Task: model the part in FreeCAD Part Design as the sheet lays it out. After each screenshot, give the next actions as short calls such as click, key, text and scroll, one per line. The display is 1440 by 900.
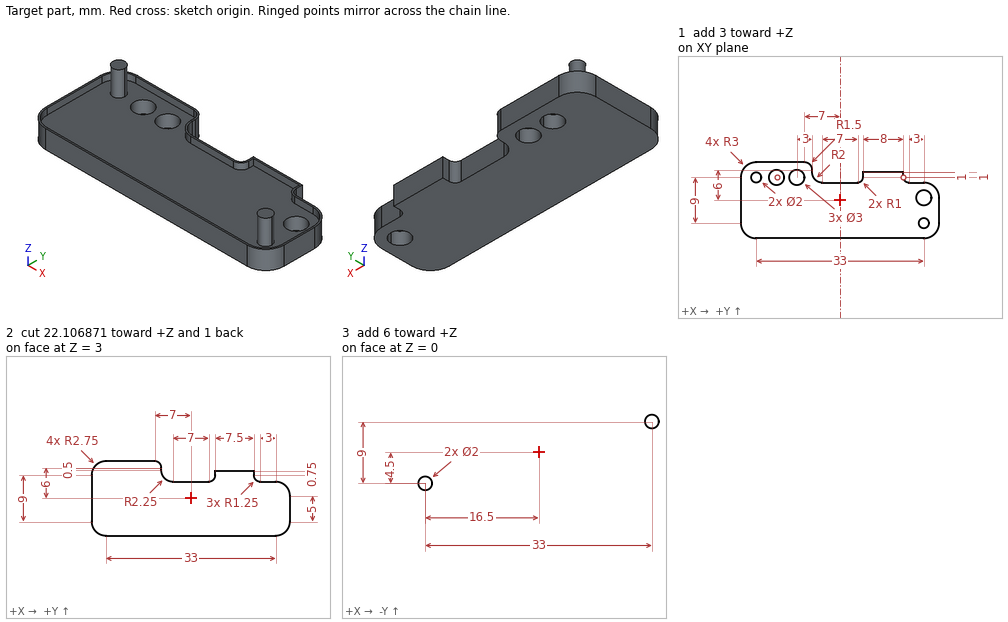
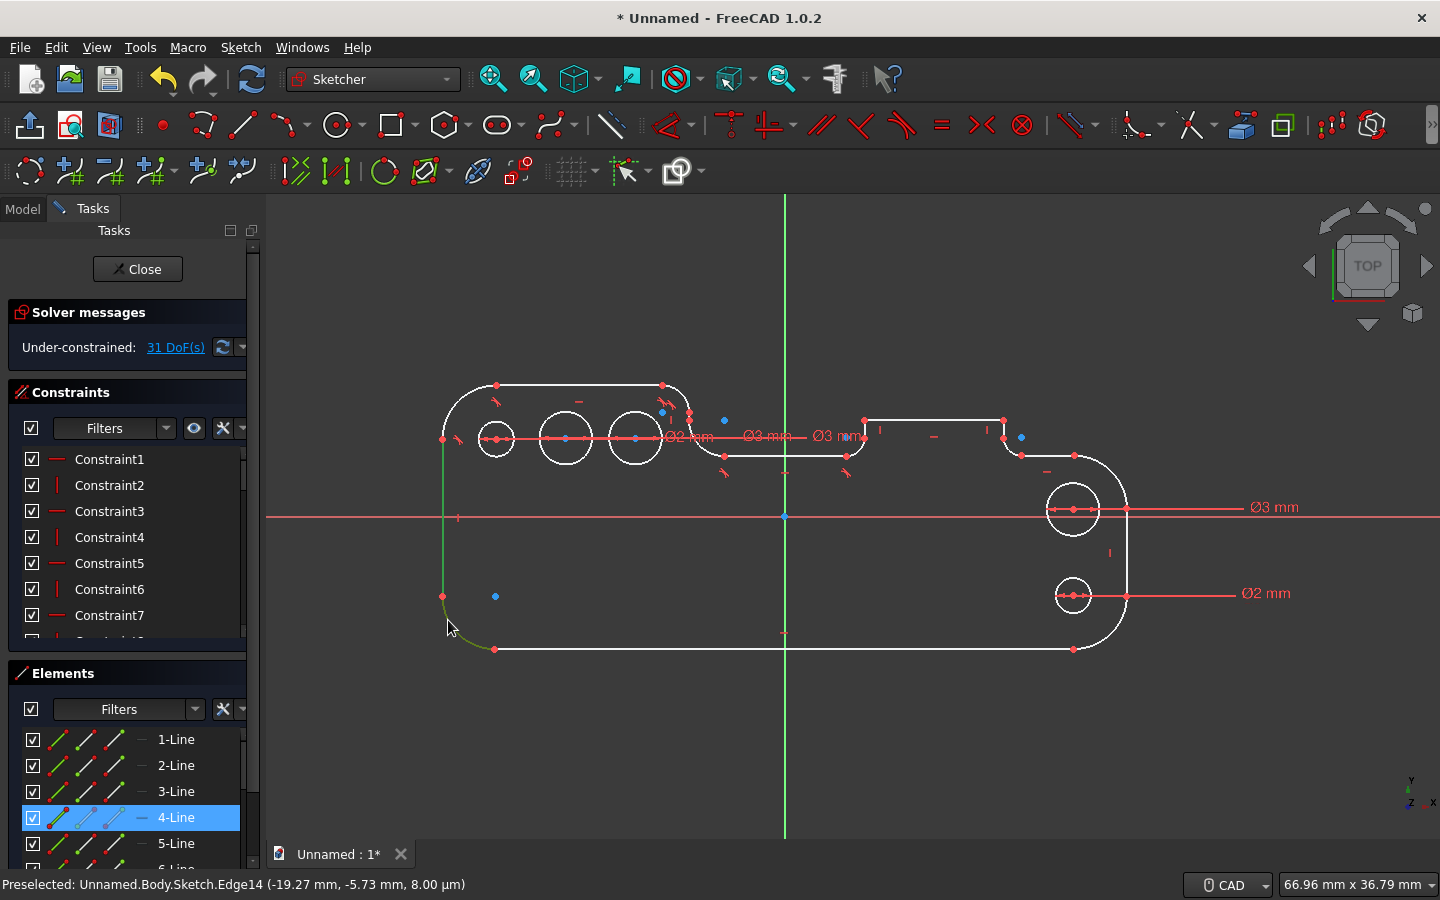
key(t)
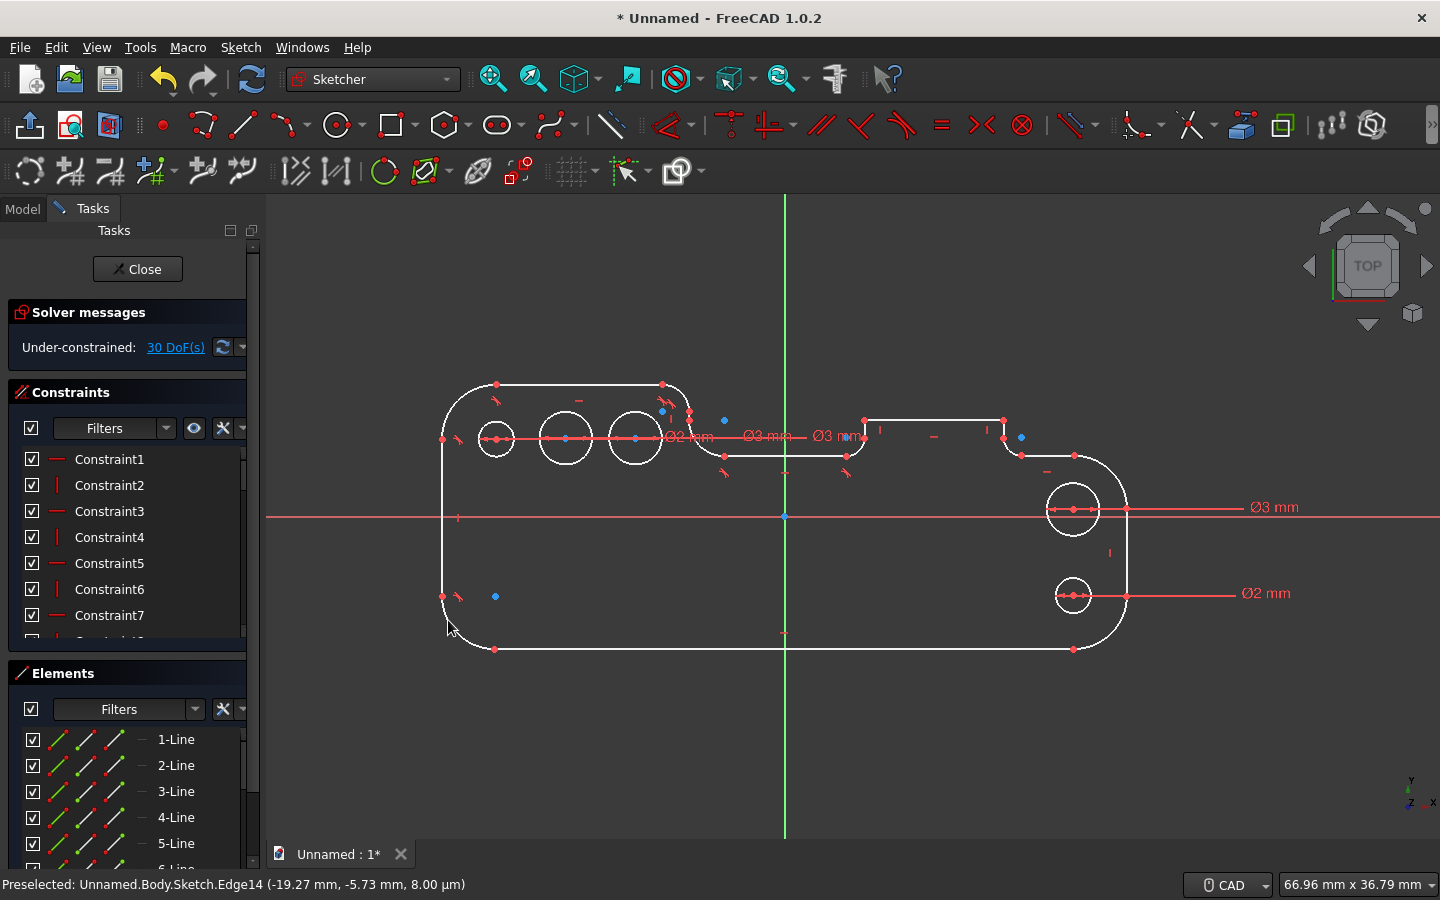
click(669, 649)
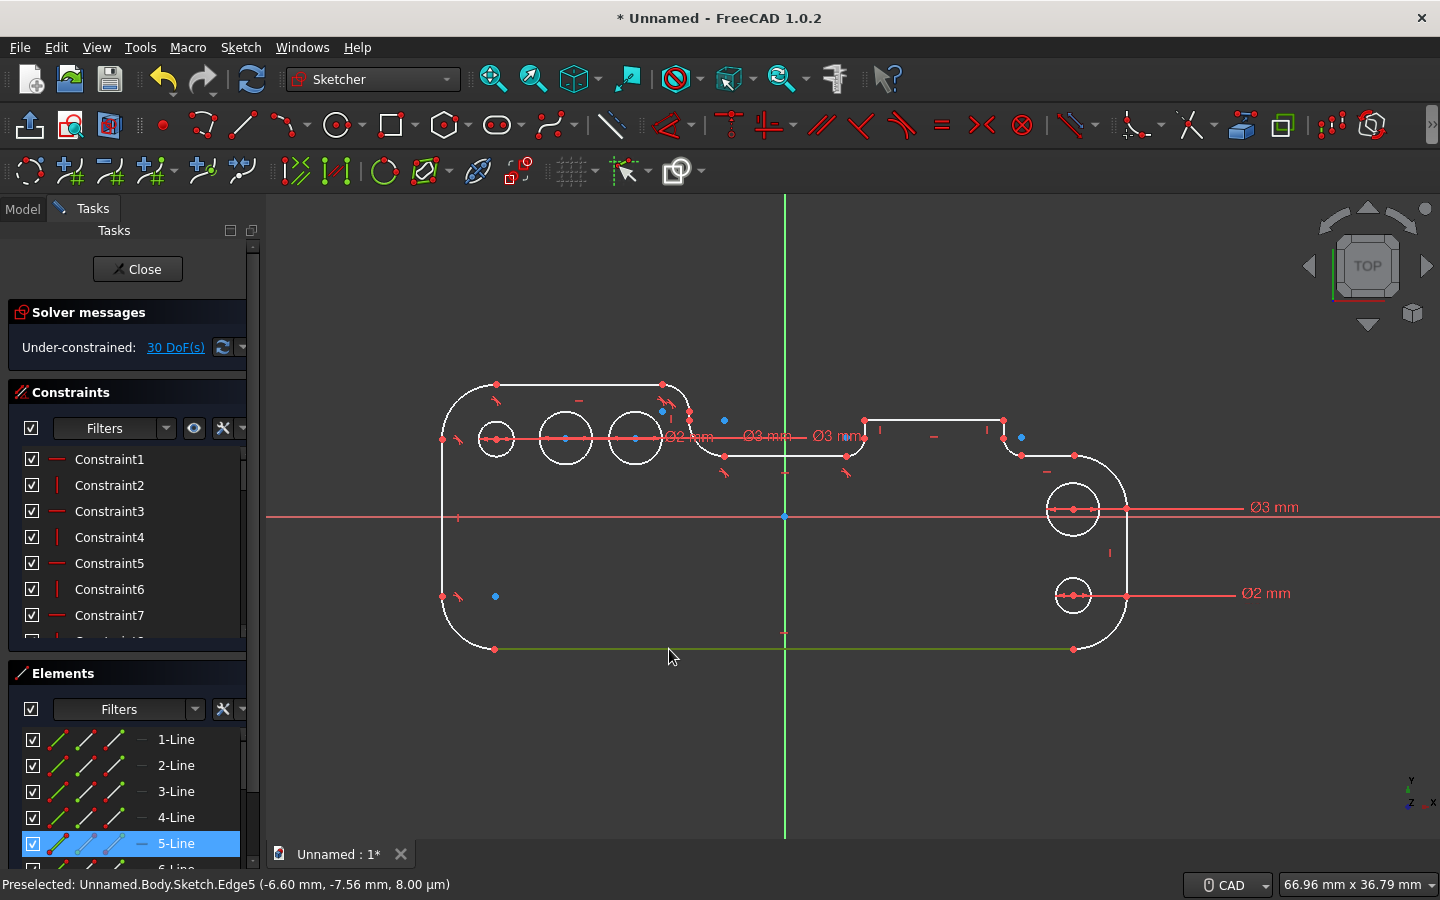
click(448, 620)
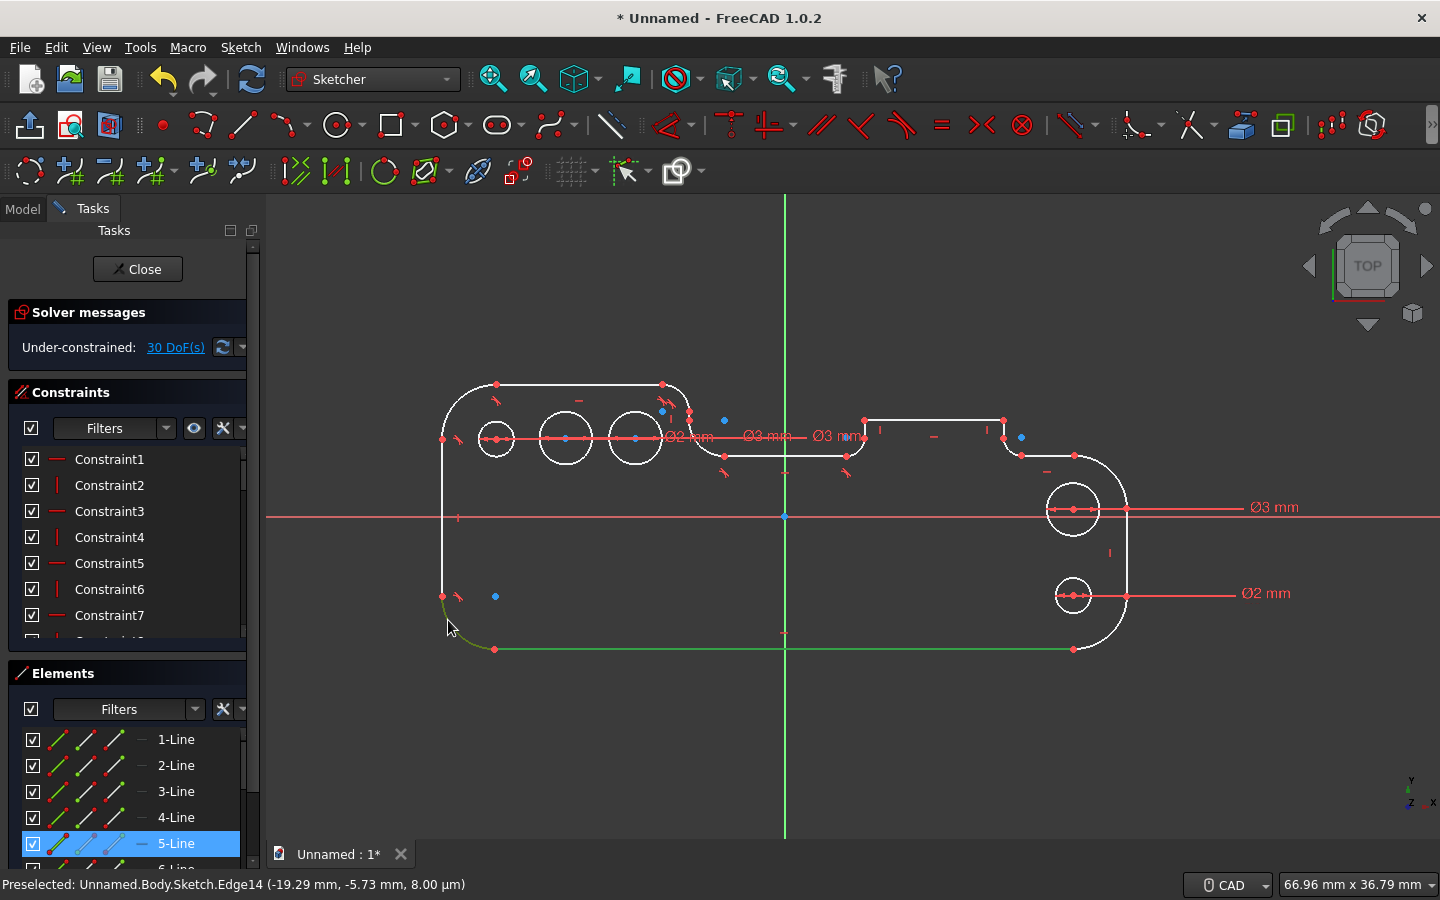
click(902, 126)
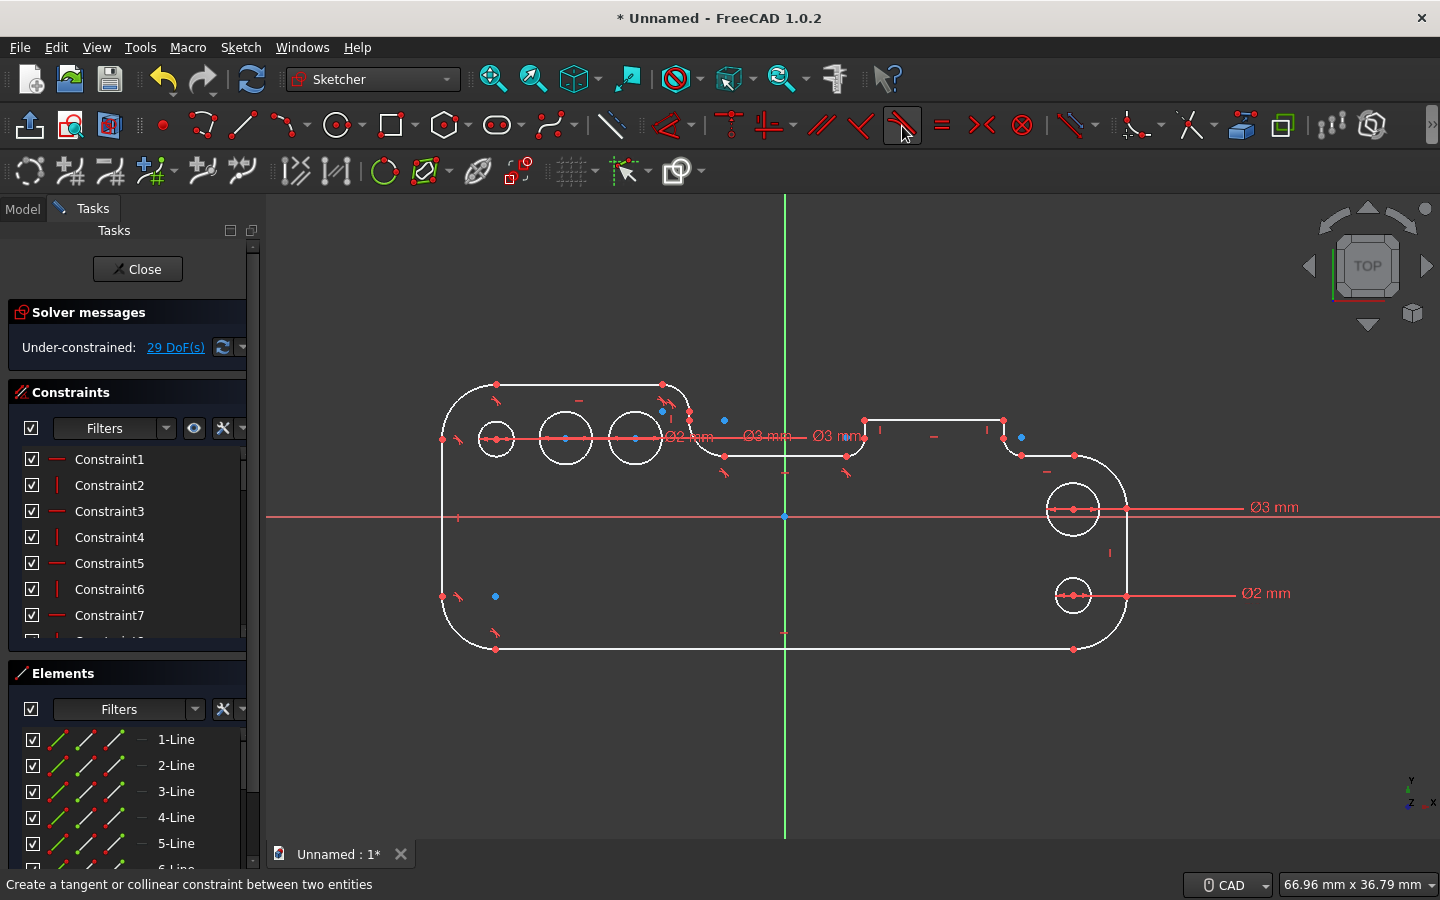
click(669, 649)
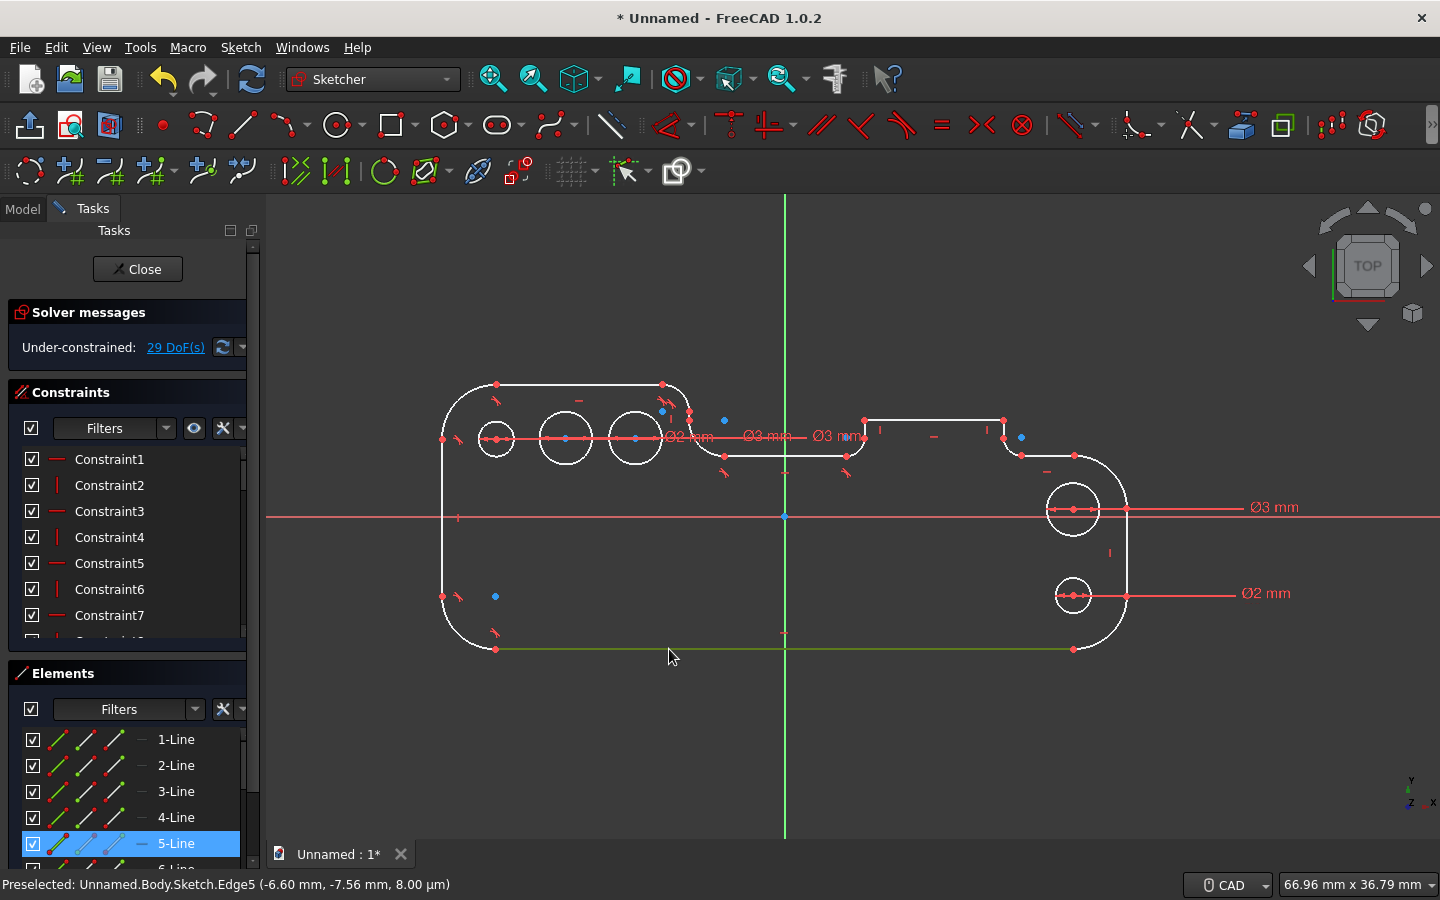
click(1098, 643)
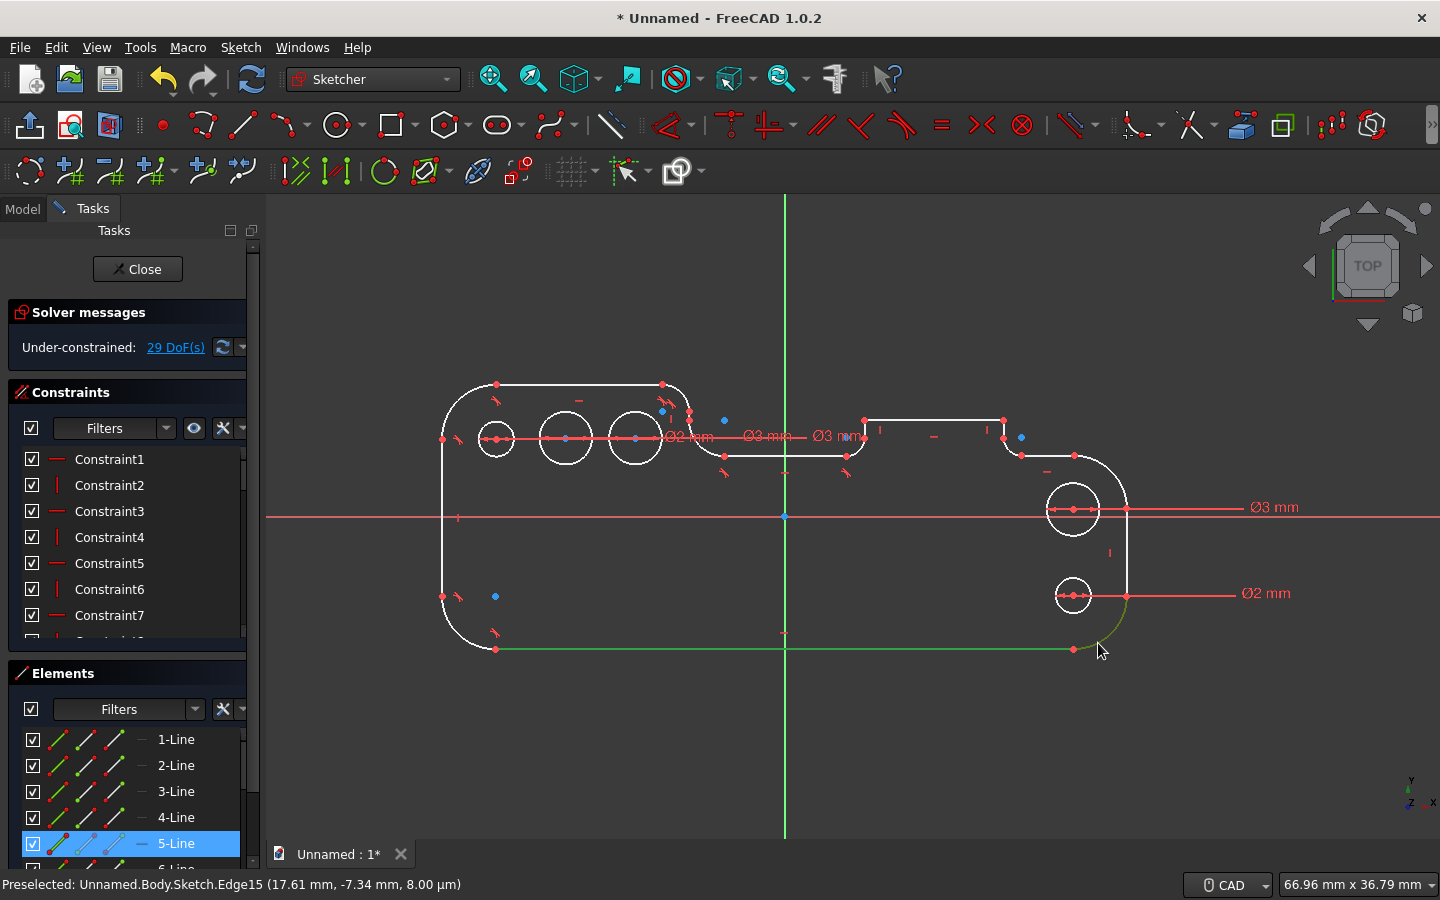
click(902, 126)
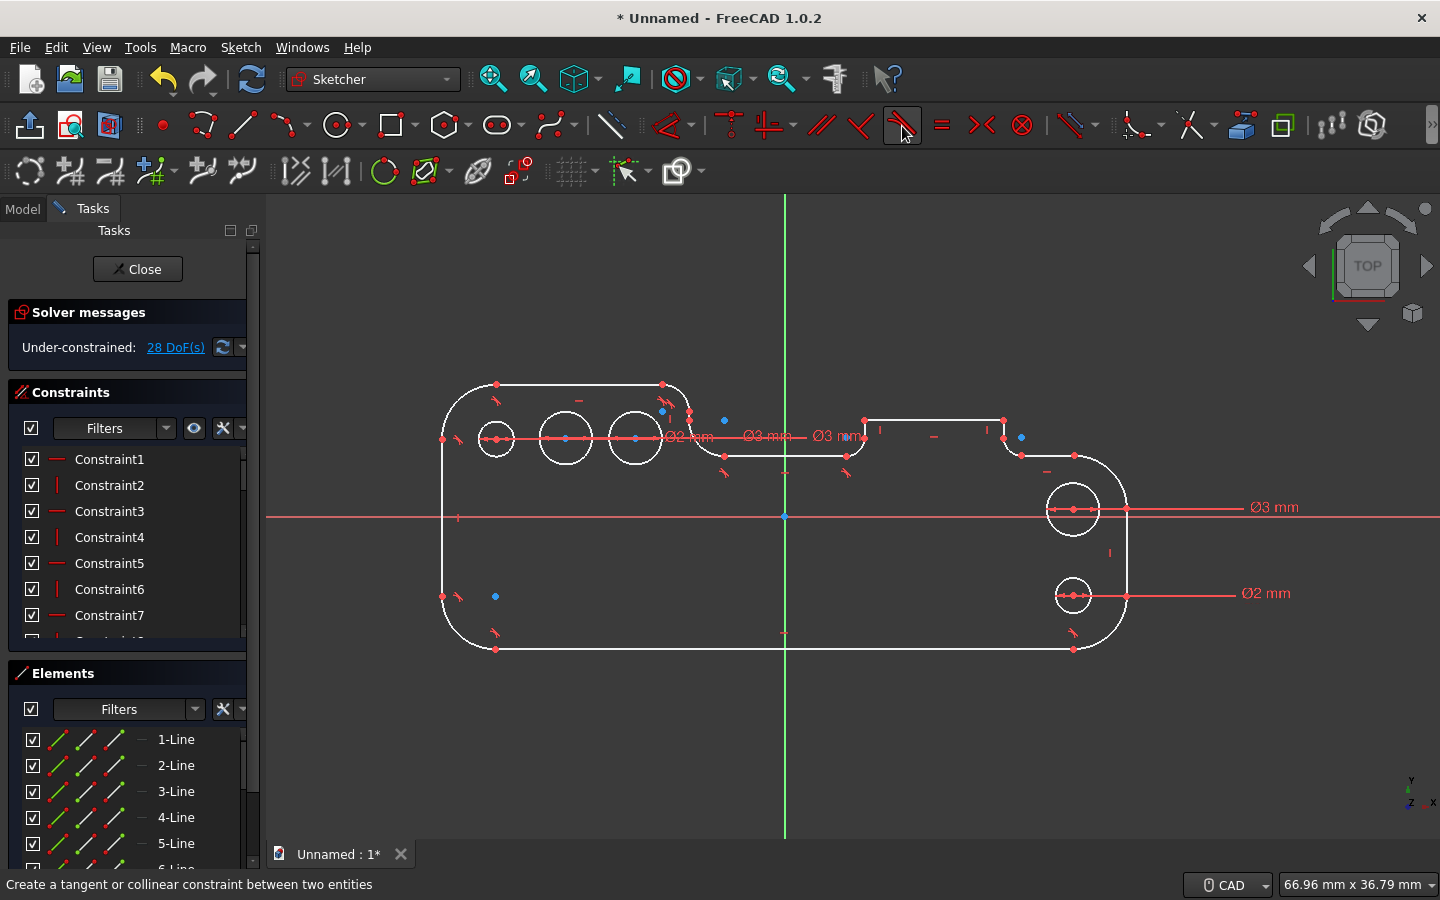
click(1127, 570)